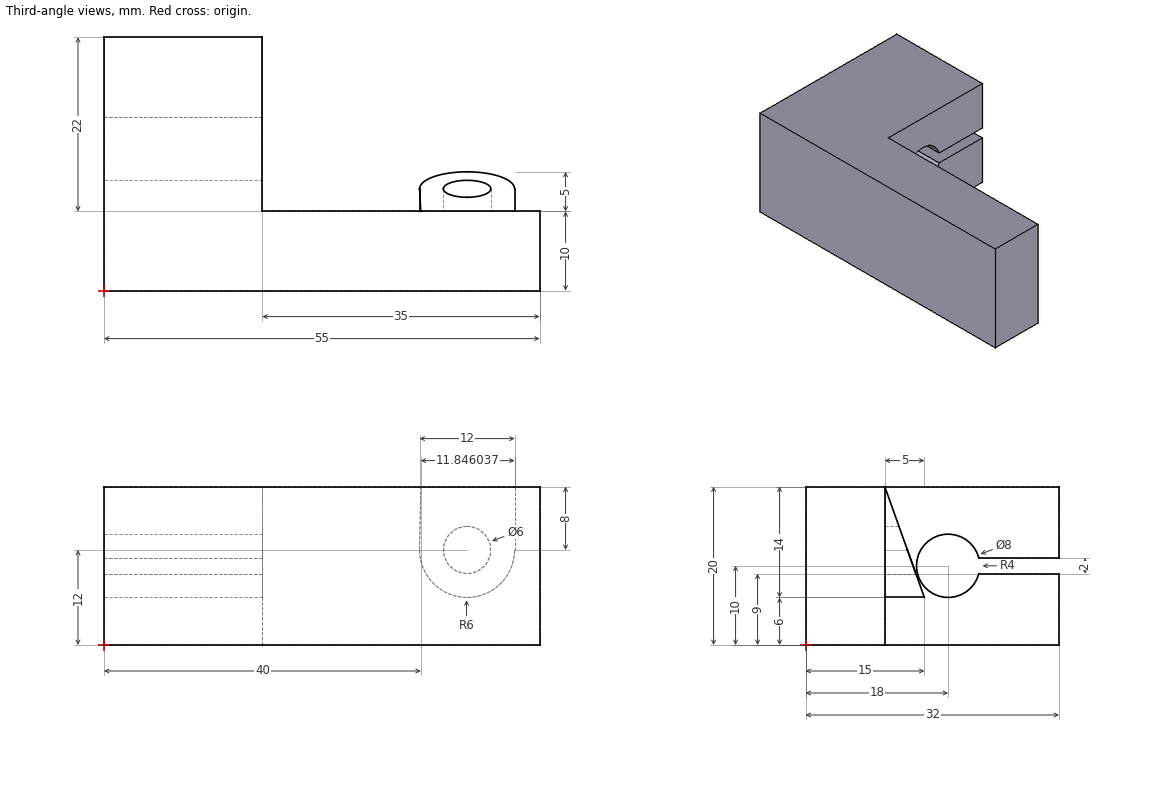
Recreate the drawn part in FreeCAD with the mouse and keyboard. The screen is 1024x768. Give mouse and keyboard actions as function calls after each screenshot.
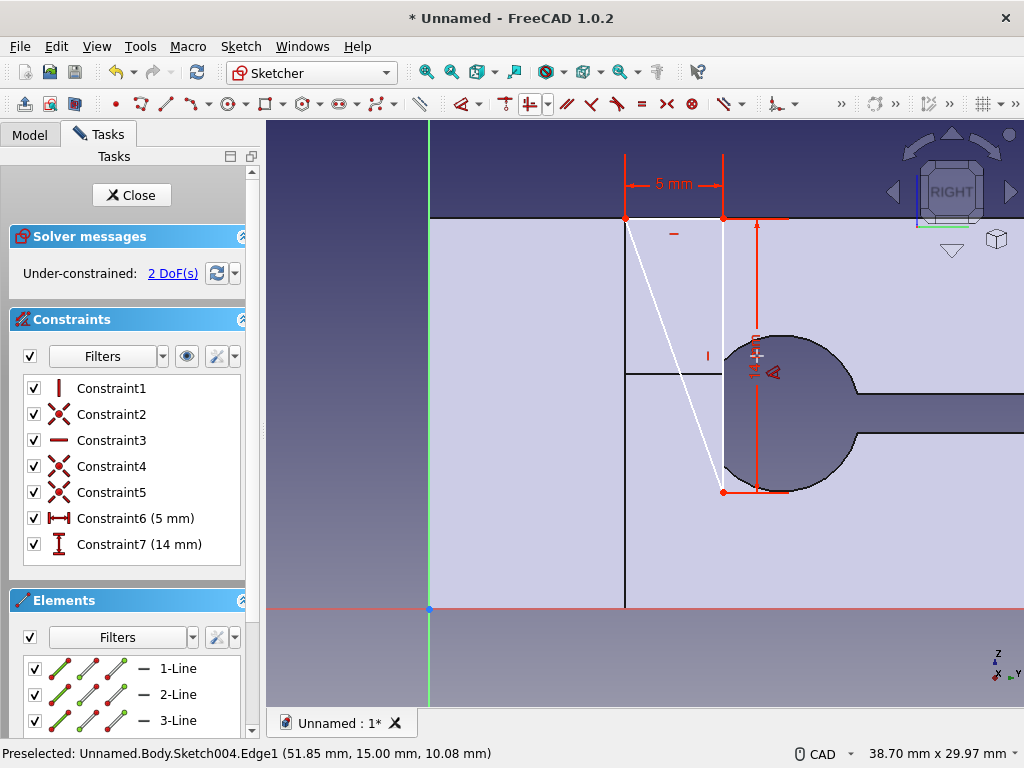
click(723, 493)
click(757, 551)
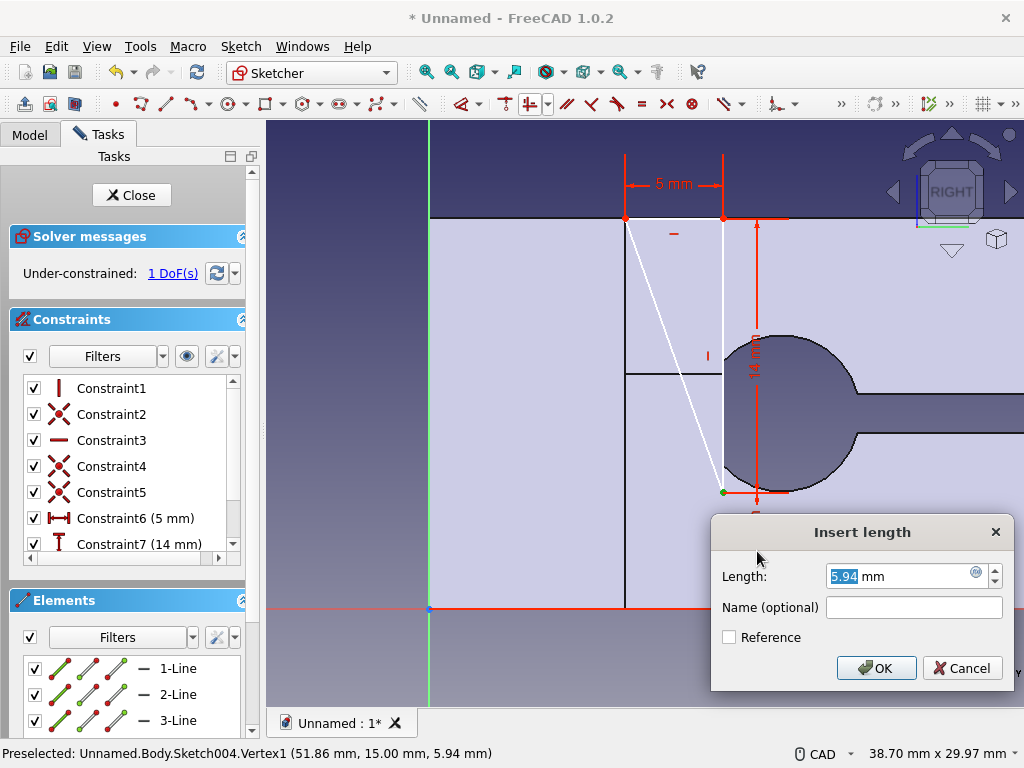
text(6)
key(Return)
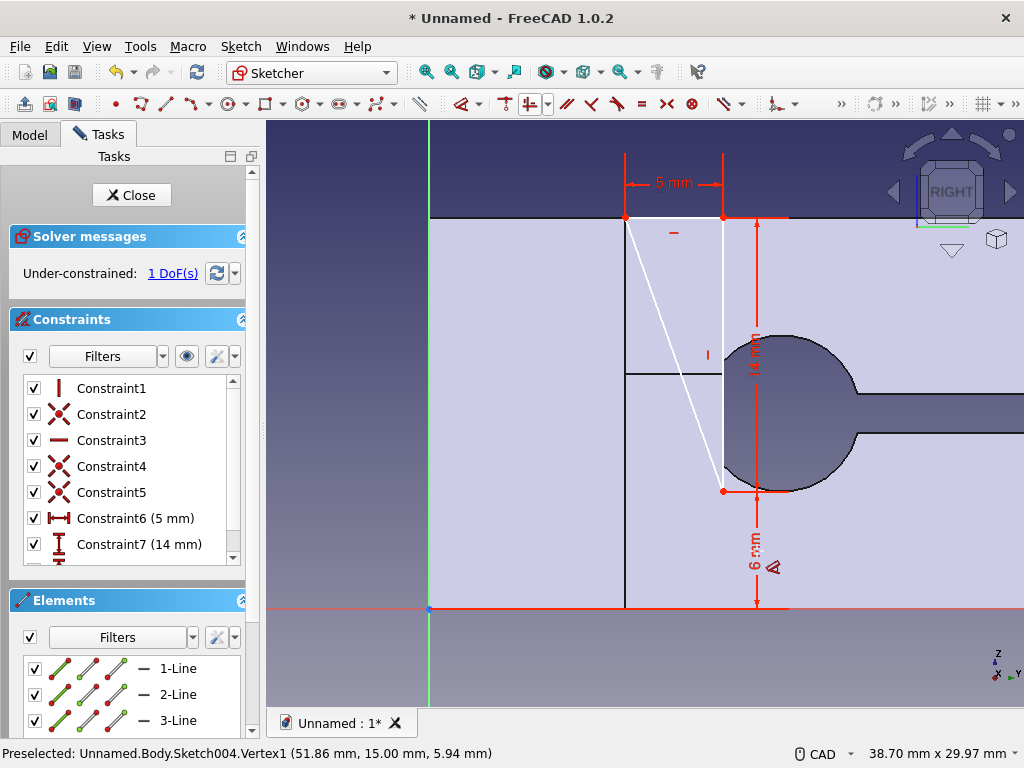
click(723, 492)
click(576, 643)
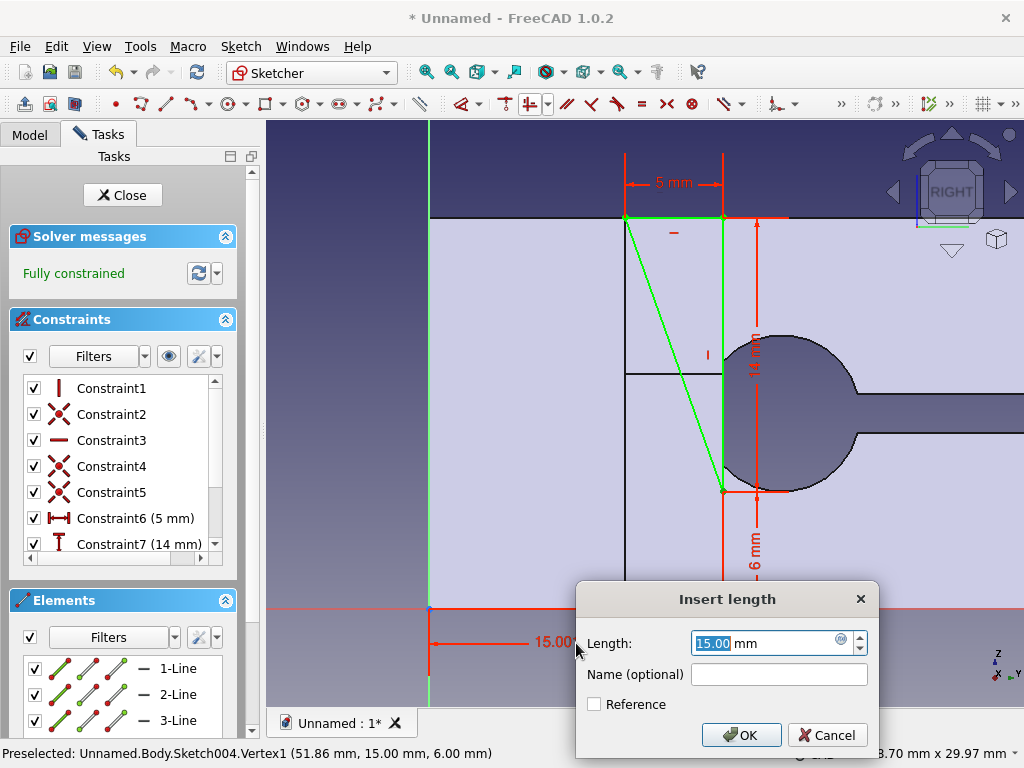
text(15)
key(Return)
key(Escape)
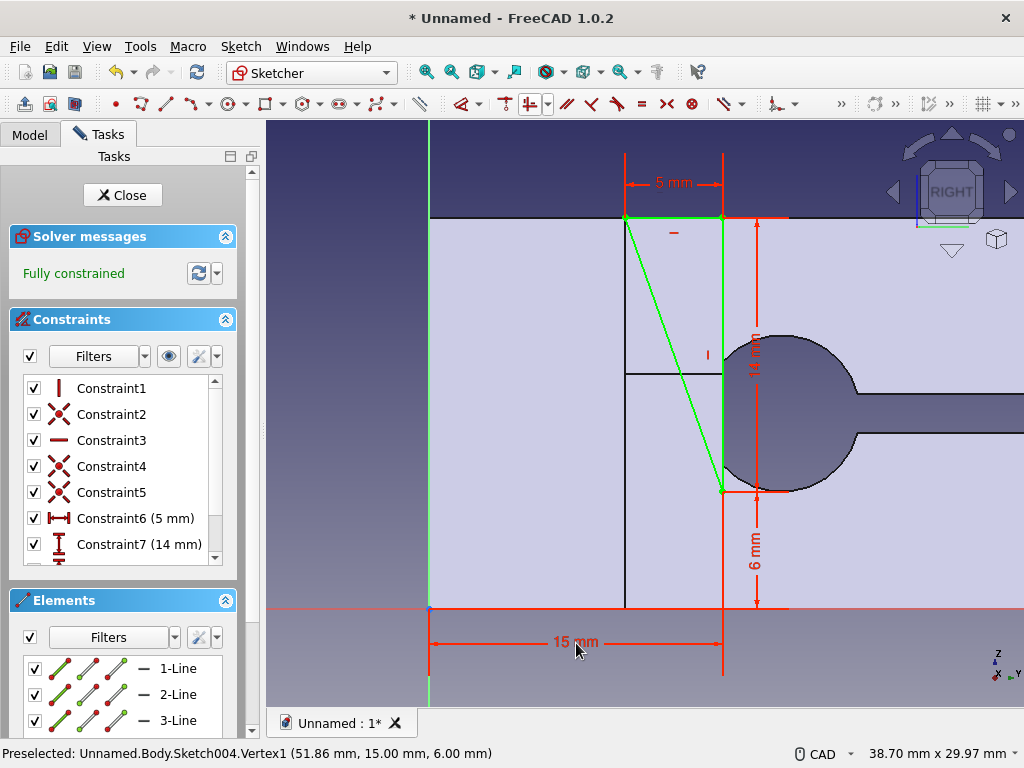
click(123, 195)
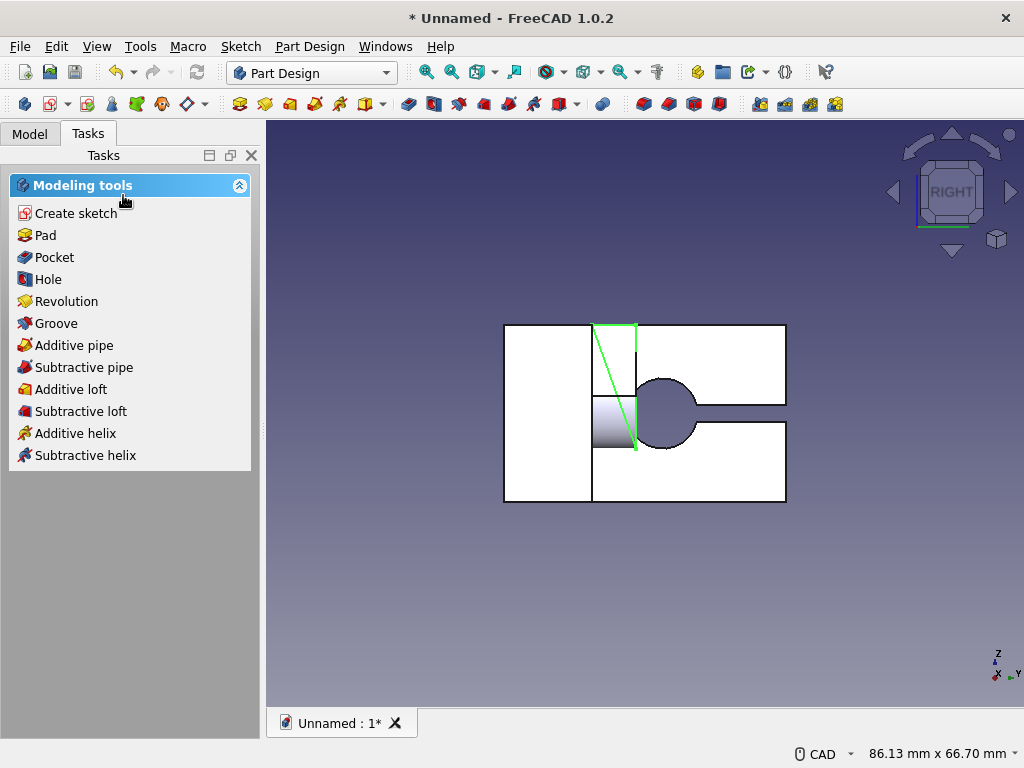
click(409, 104)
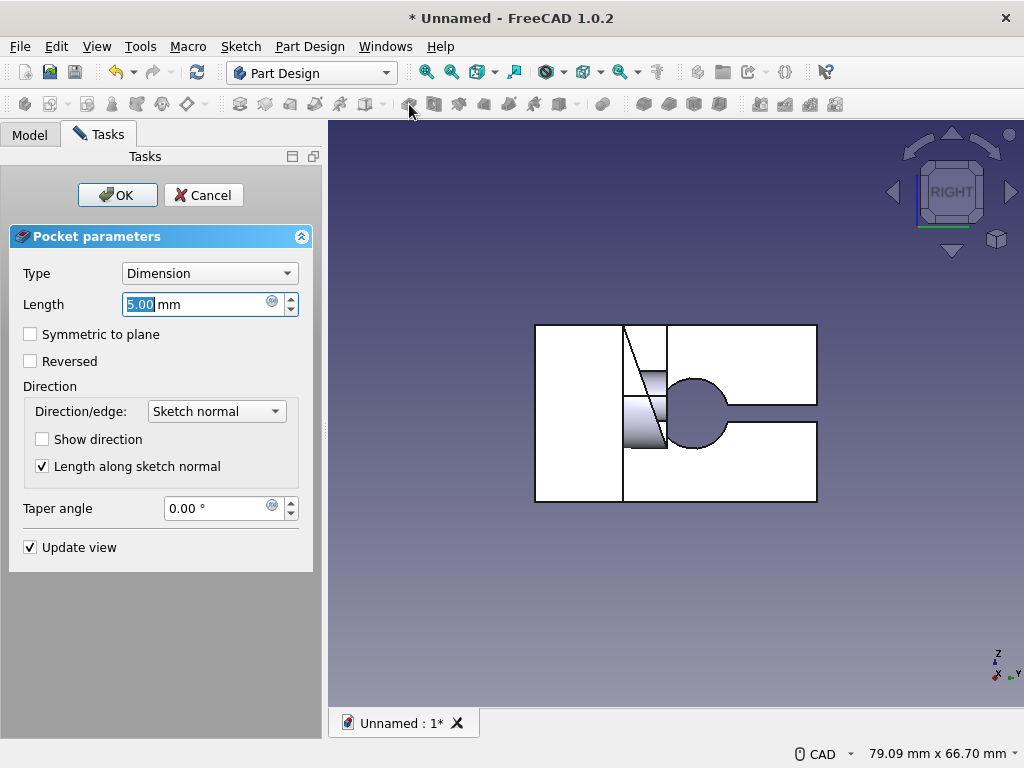
text(12)
key(Tab)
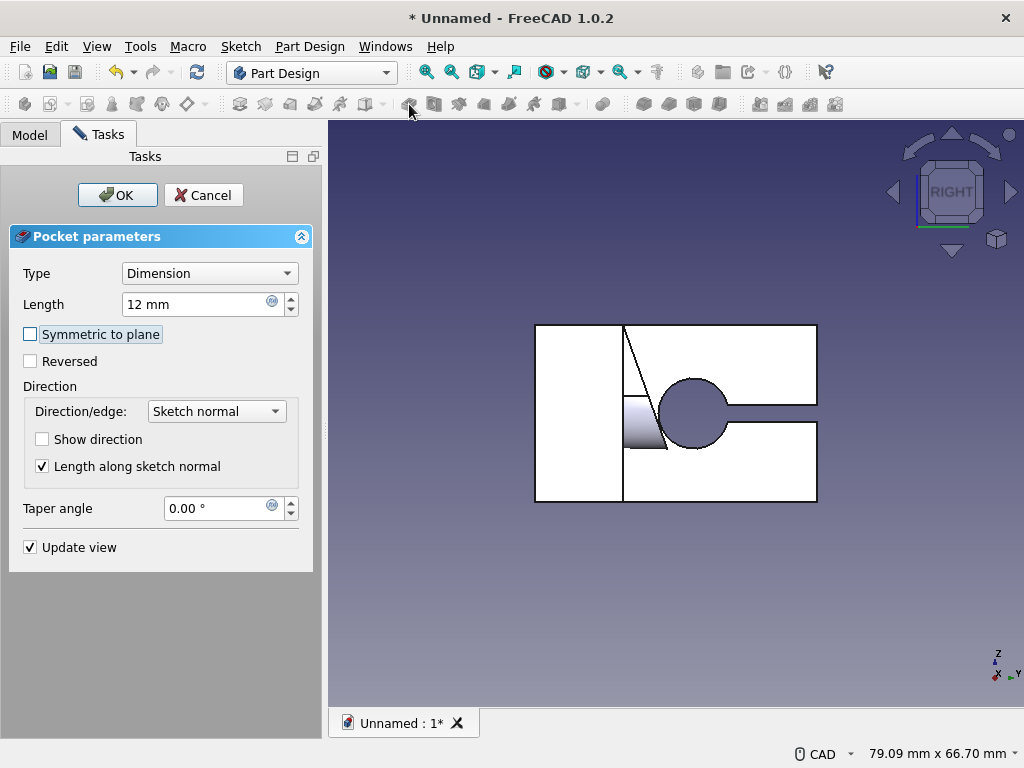
click(118, 195)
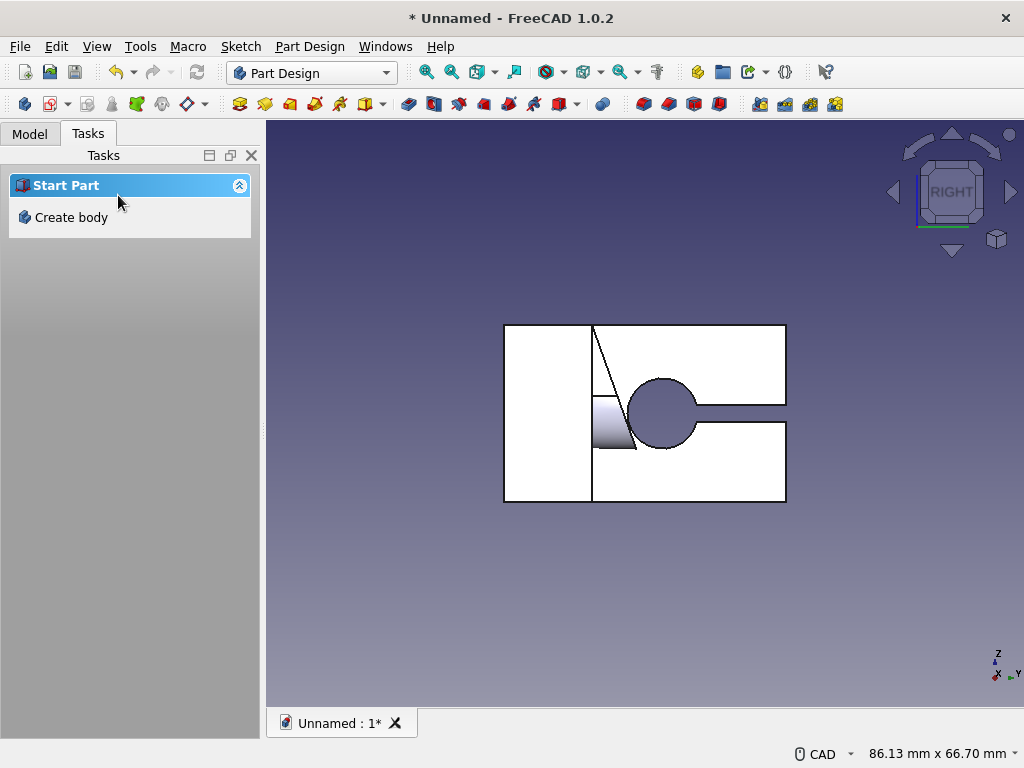
key(0)